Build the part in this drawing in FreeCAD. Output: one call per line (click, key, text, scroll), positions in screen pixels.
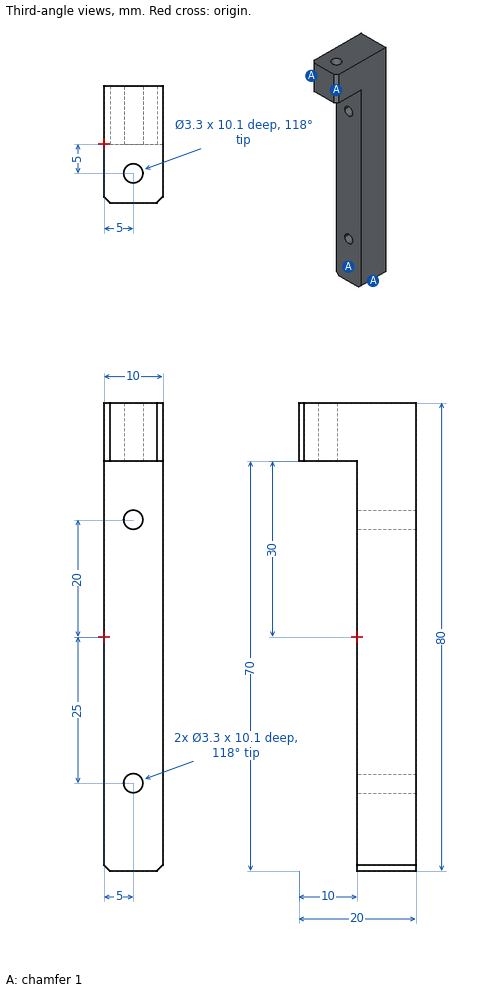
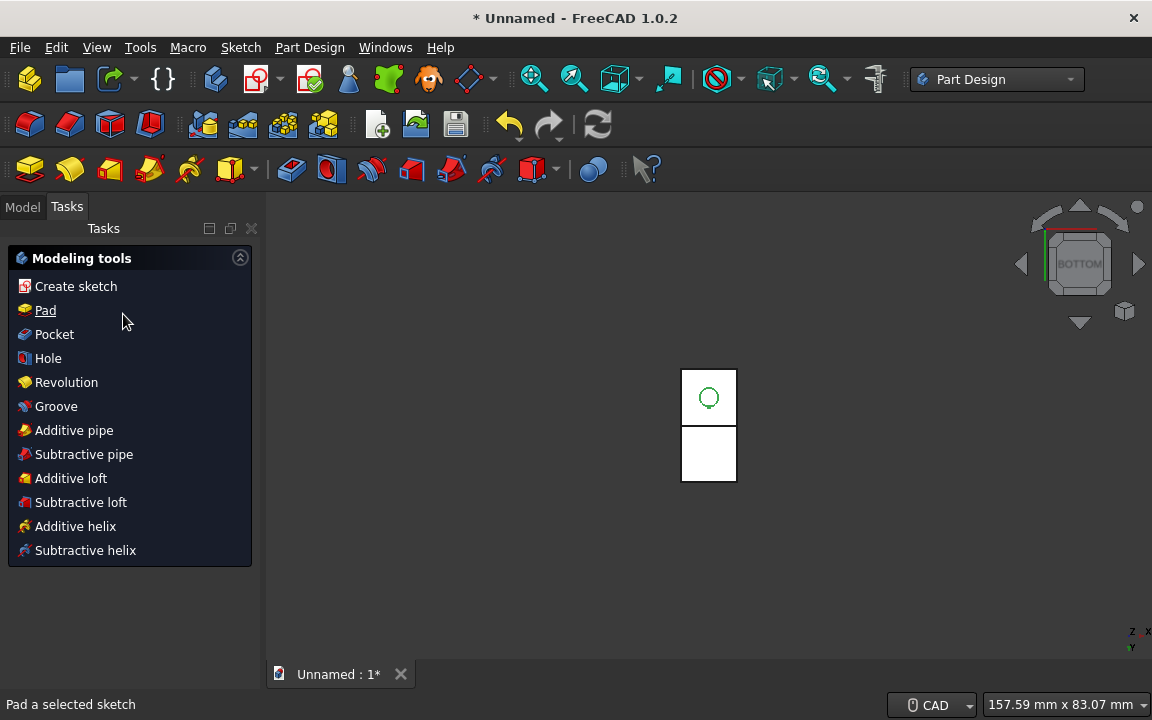
click(332, 170)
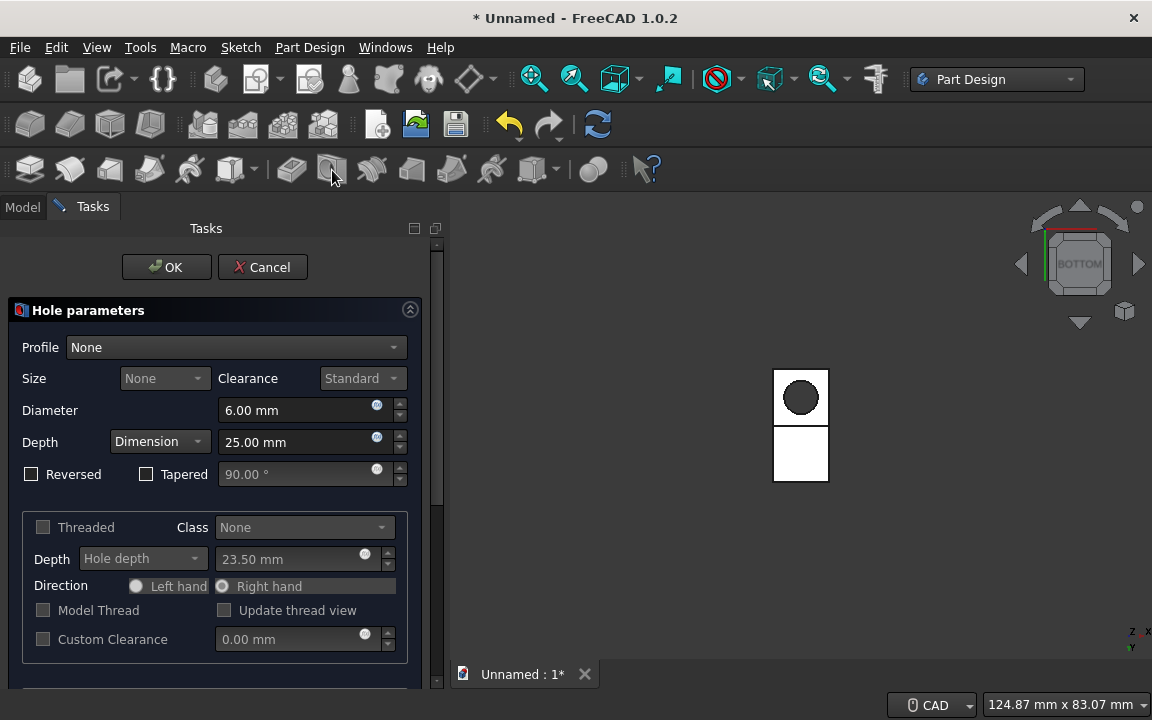
triple_click(305, 410)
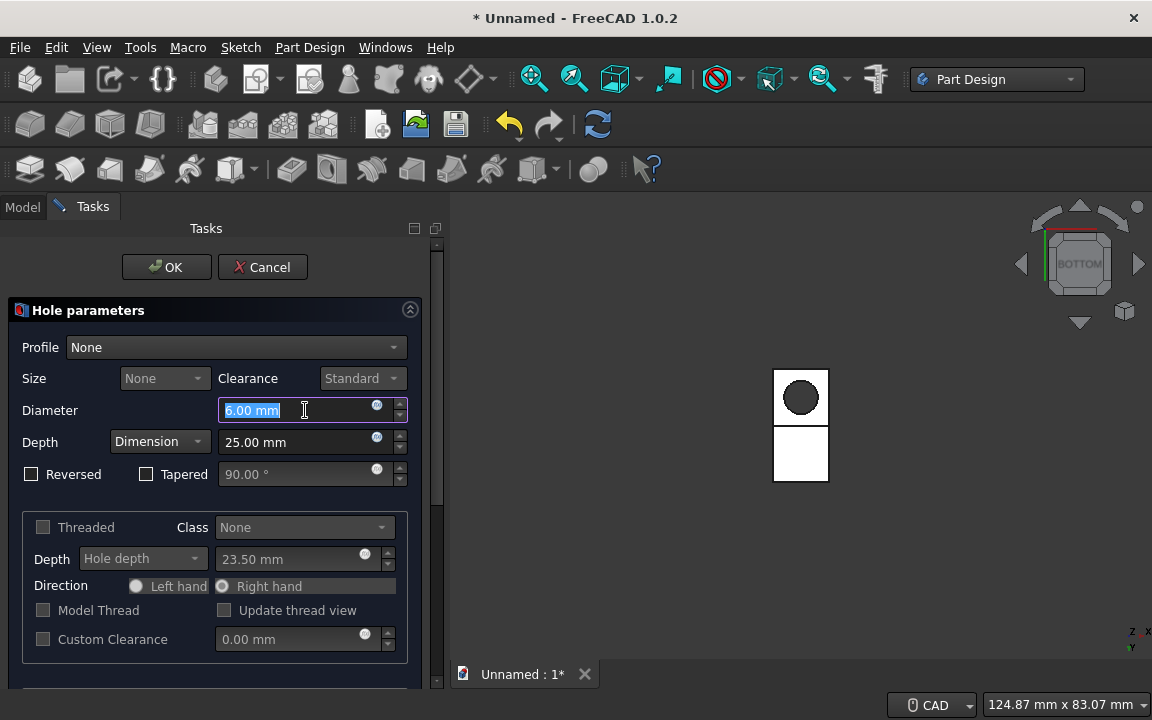
text(3.3)
key(Tab)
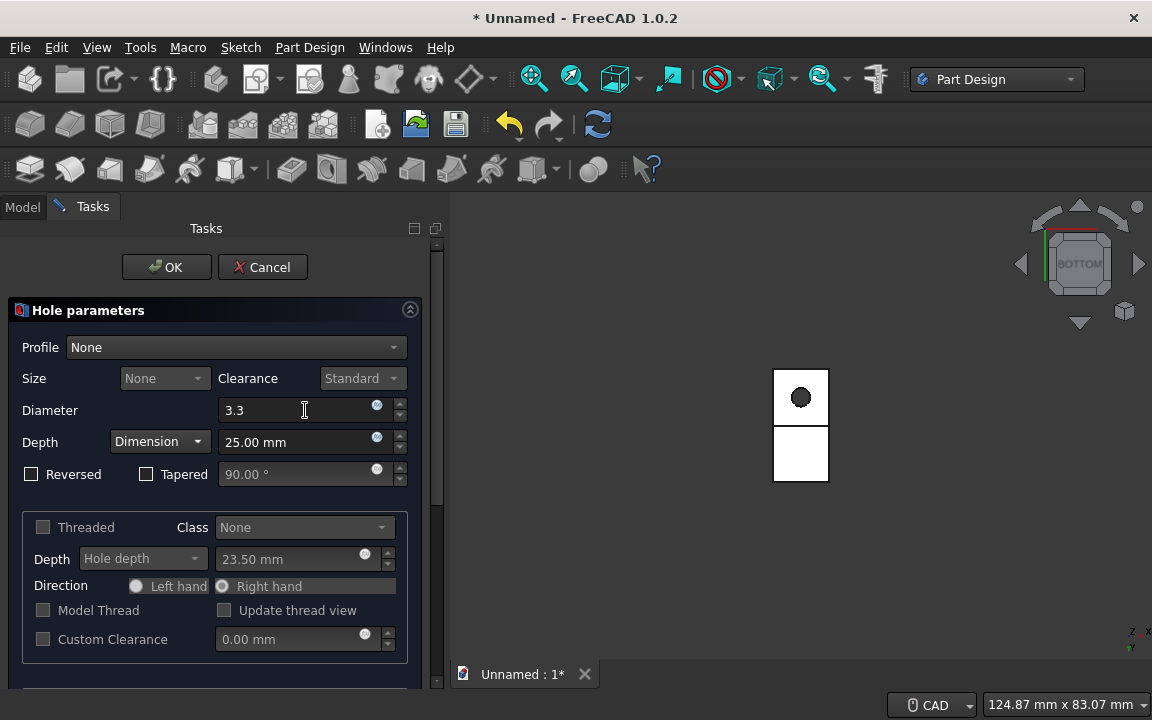
triple_click(305, 442)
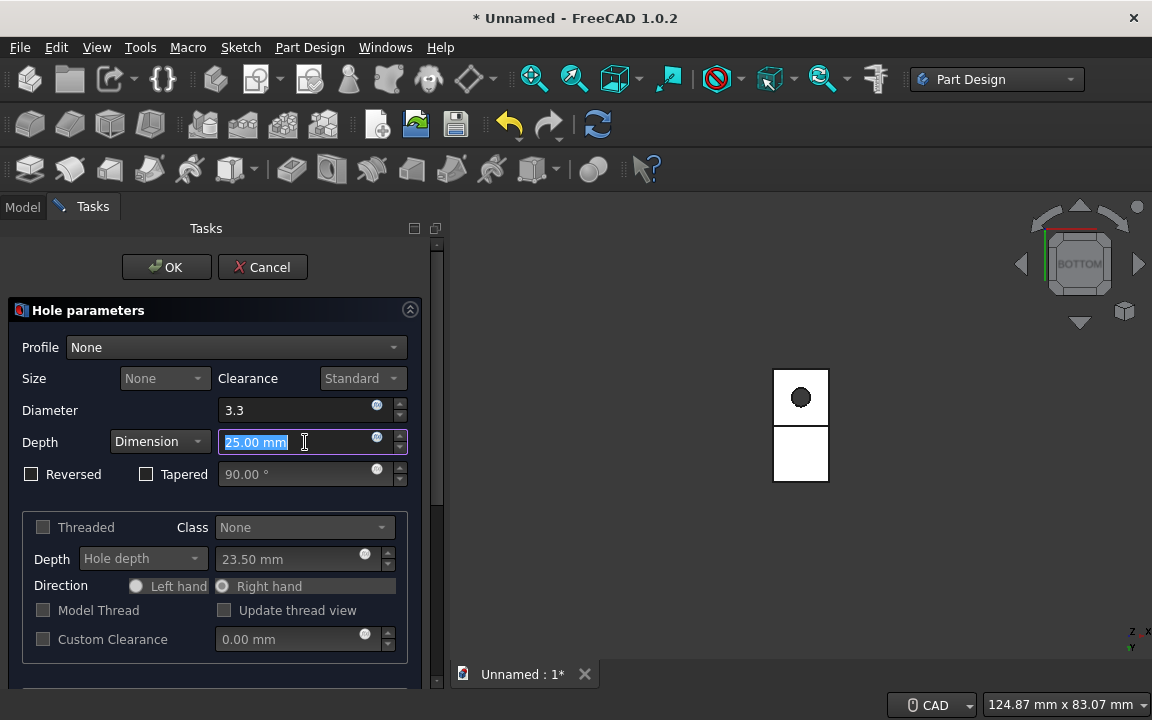
text(10.1)
key(Tab)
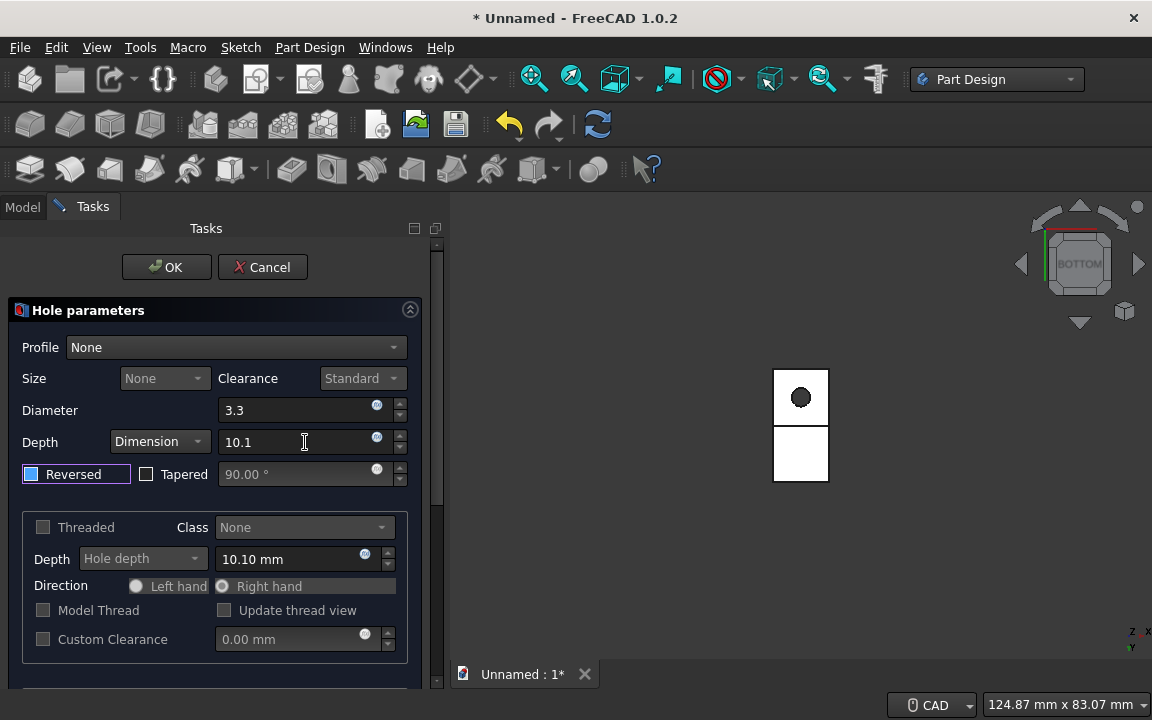
click(167, 267)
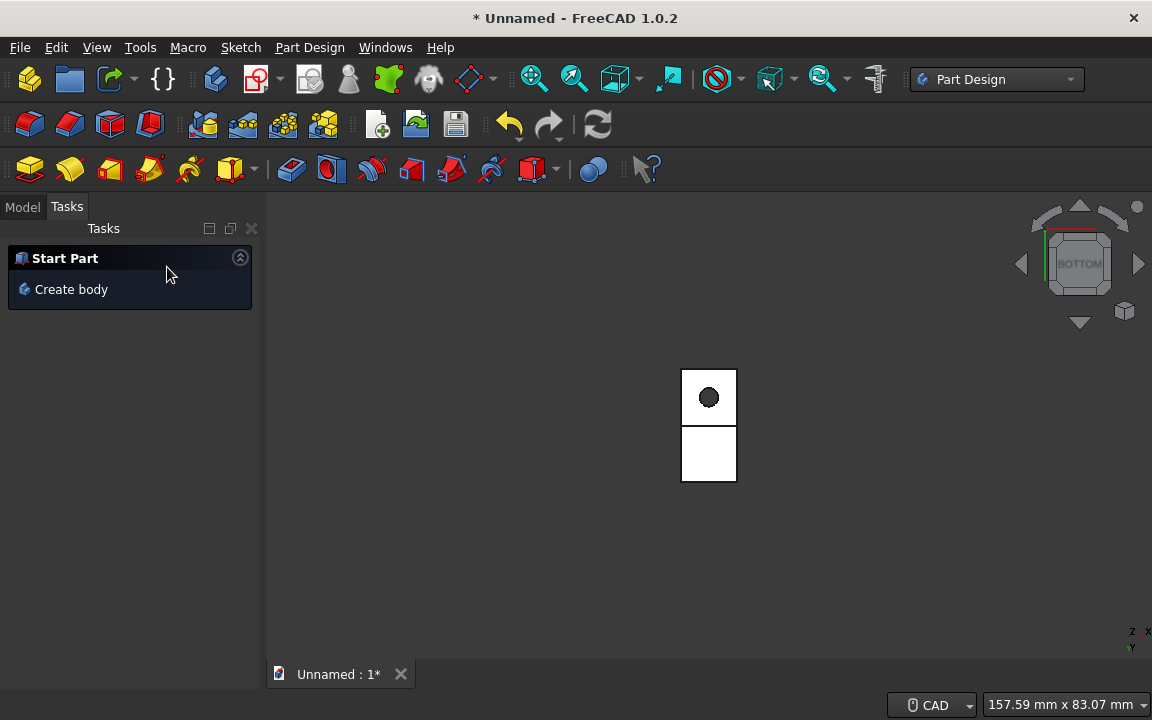
key(v)
key(f)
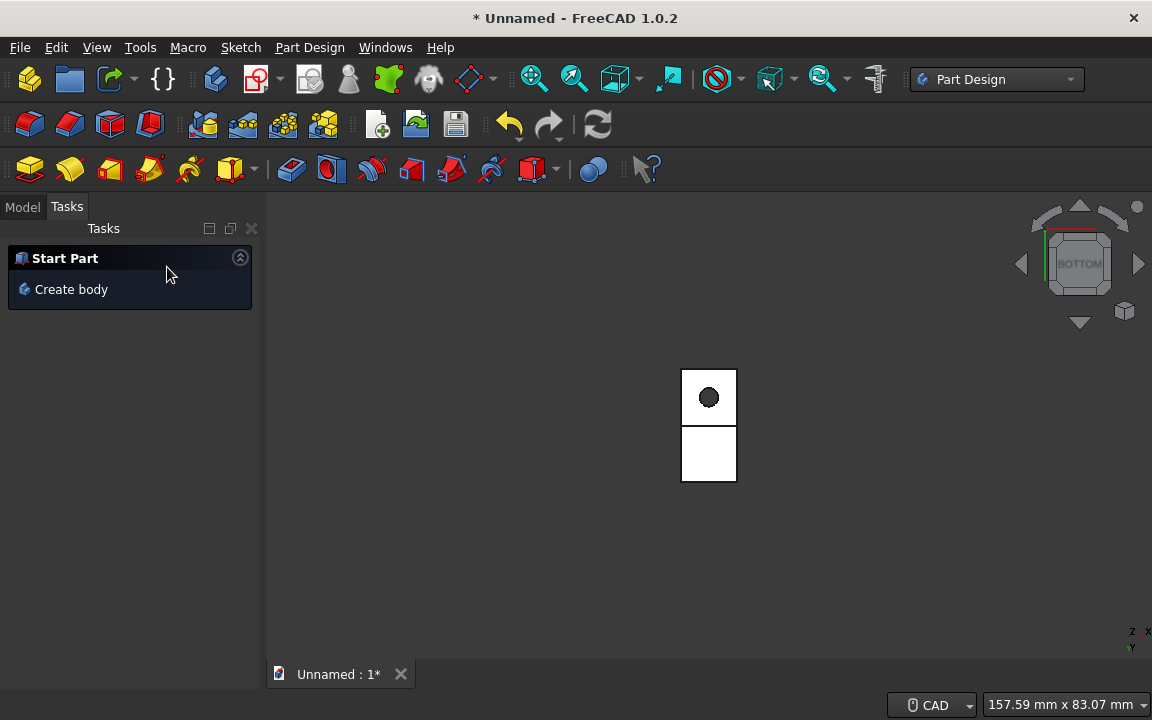
click(681, 453)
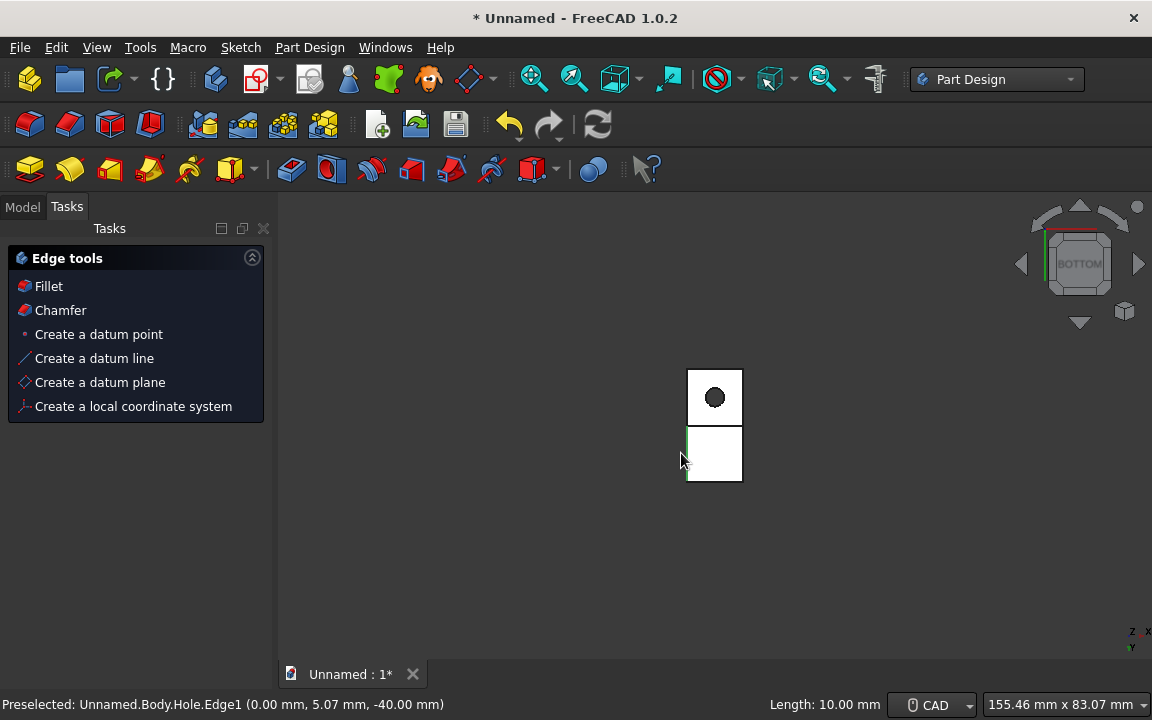
click(743, 453, ctrl)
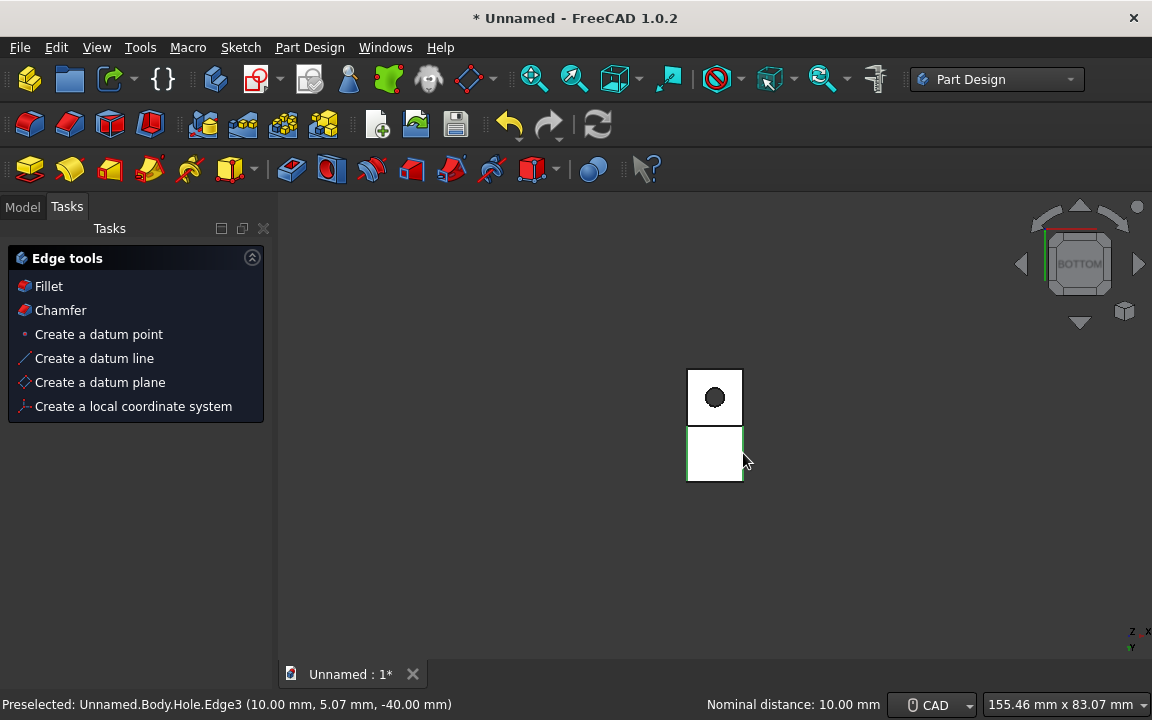
key(0)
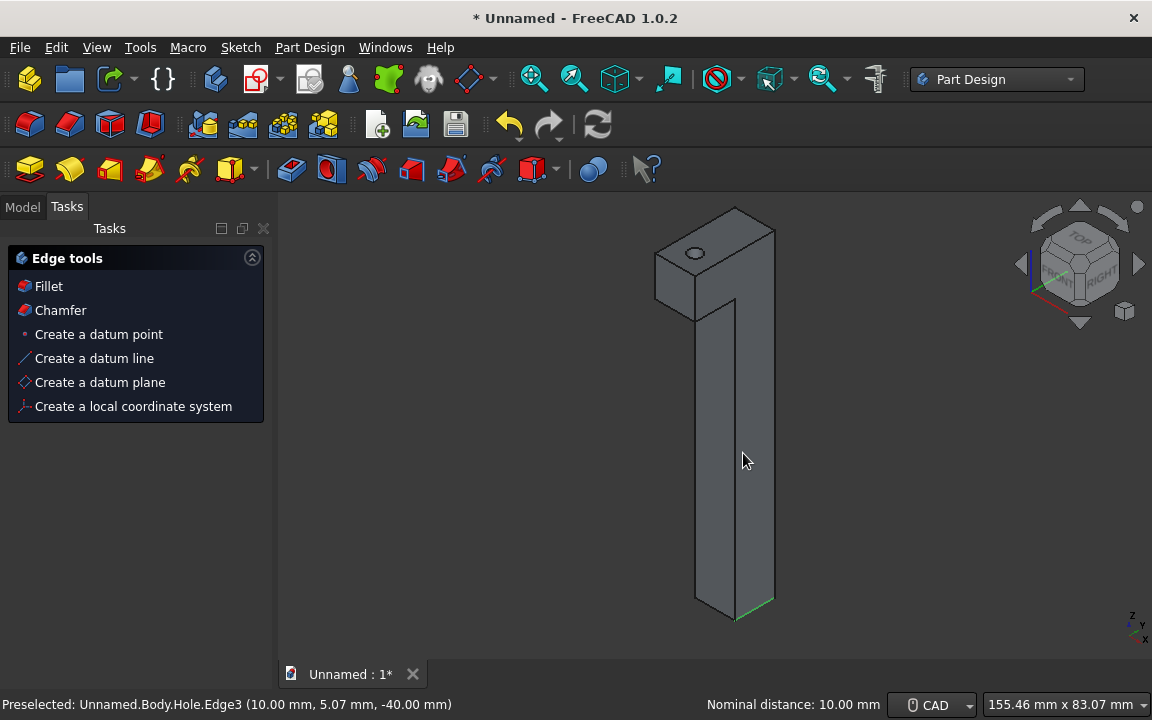
click(695, 298, ctrl)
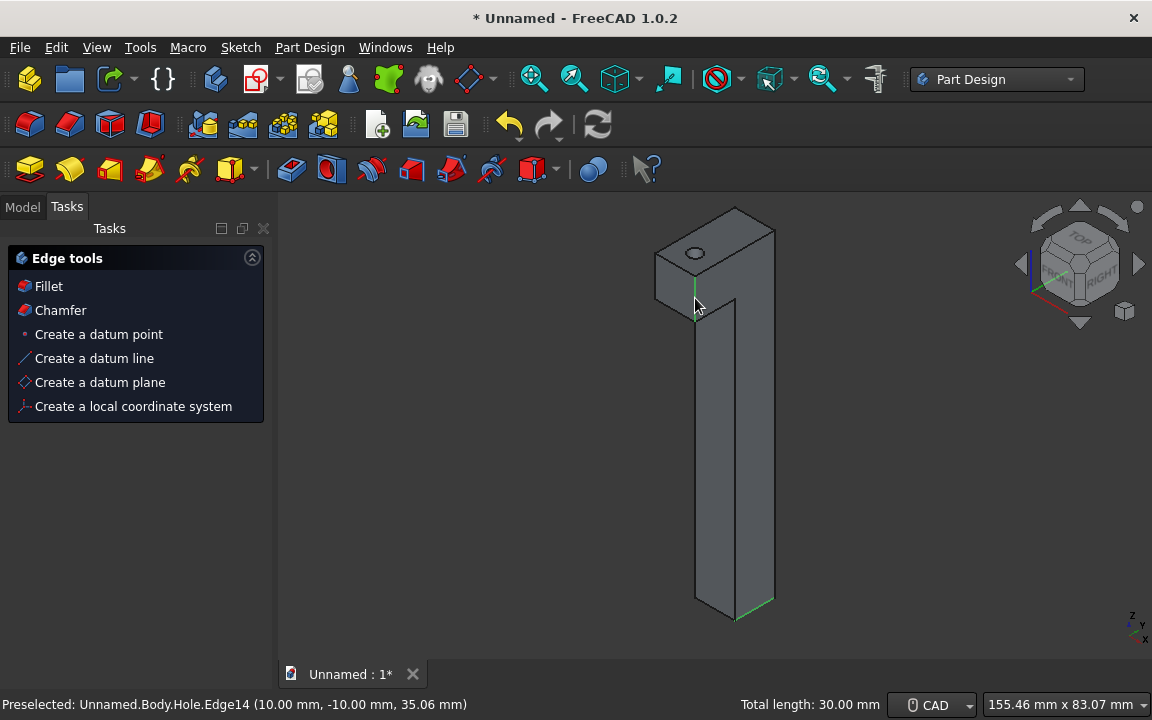
key(2)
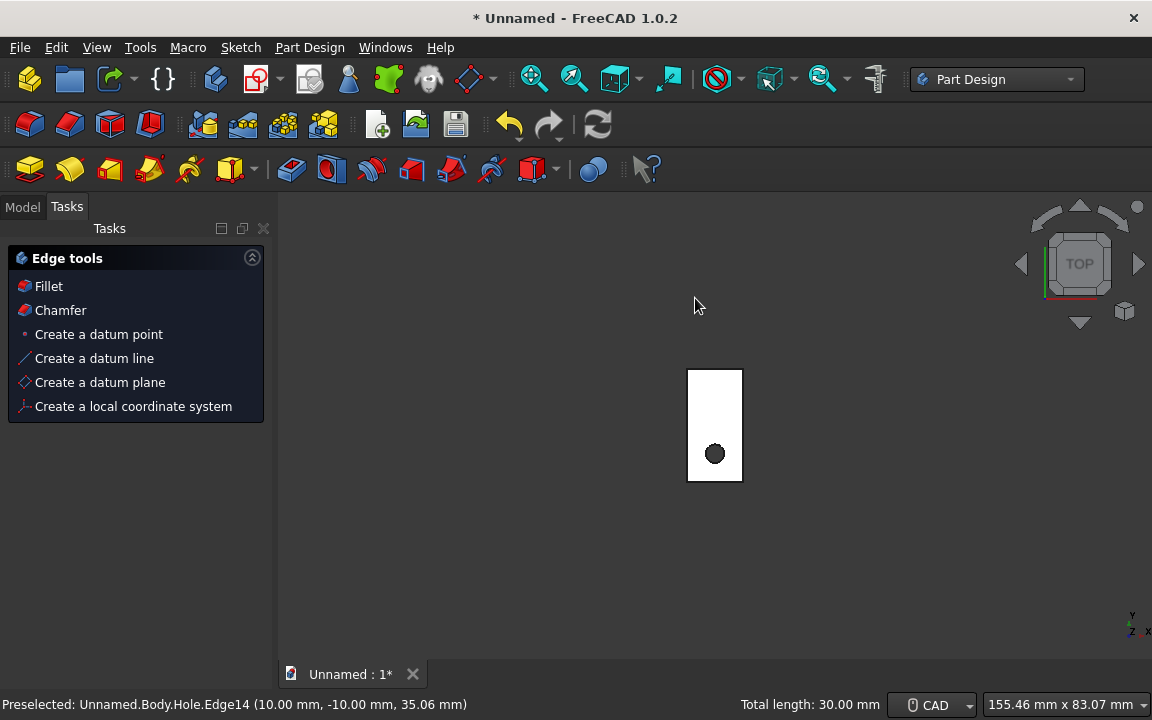
key(v)
key(f)